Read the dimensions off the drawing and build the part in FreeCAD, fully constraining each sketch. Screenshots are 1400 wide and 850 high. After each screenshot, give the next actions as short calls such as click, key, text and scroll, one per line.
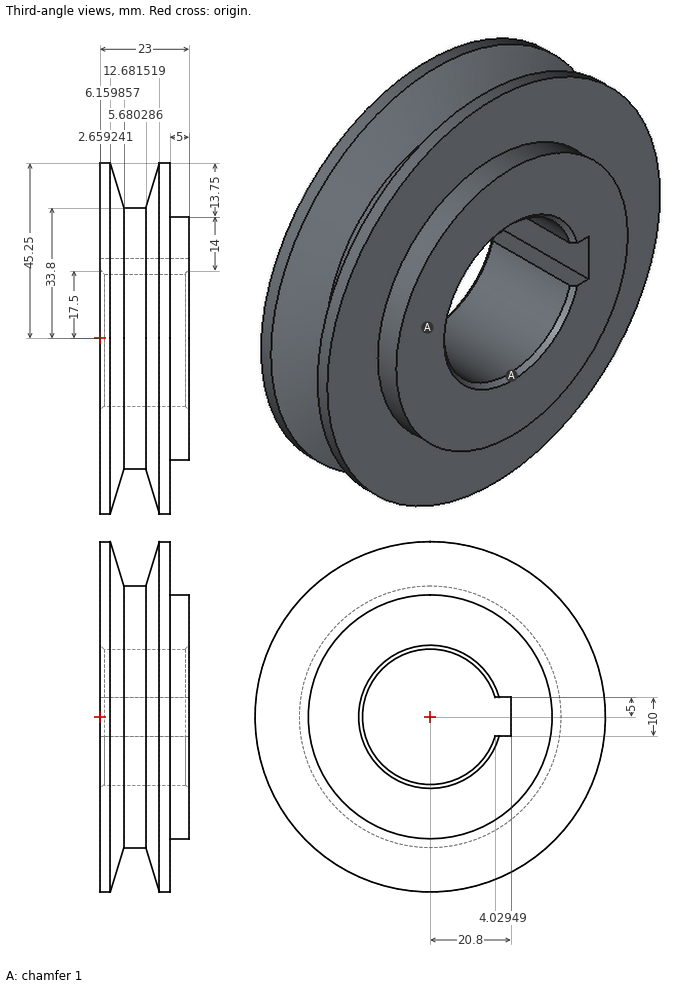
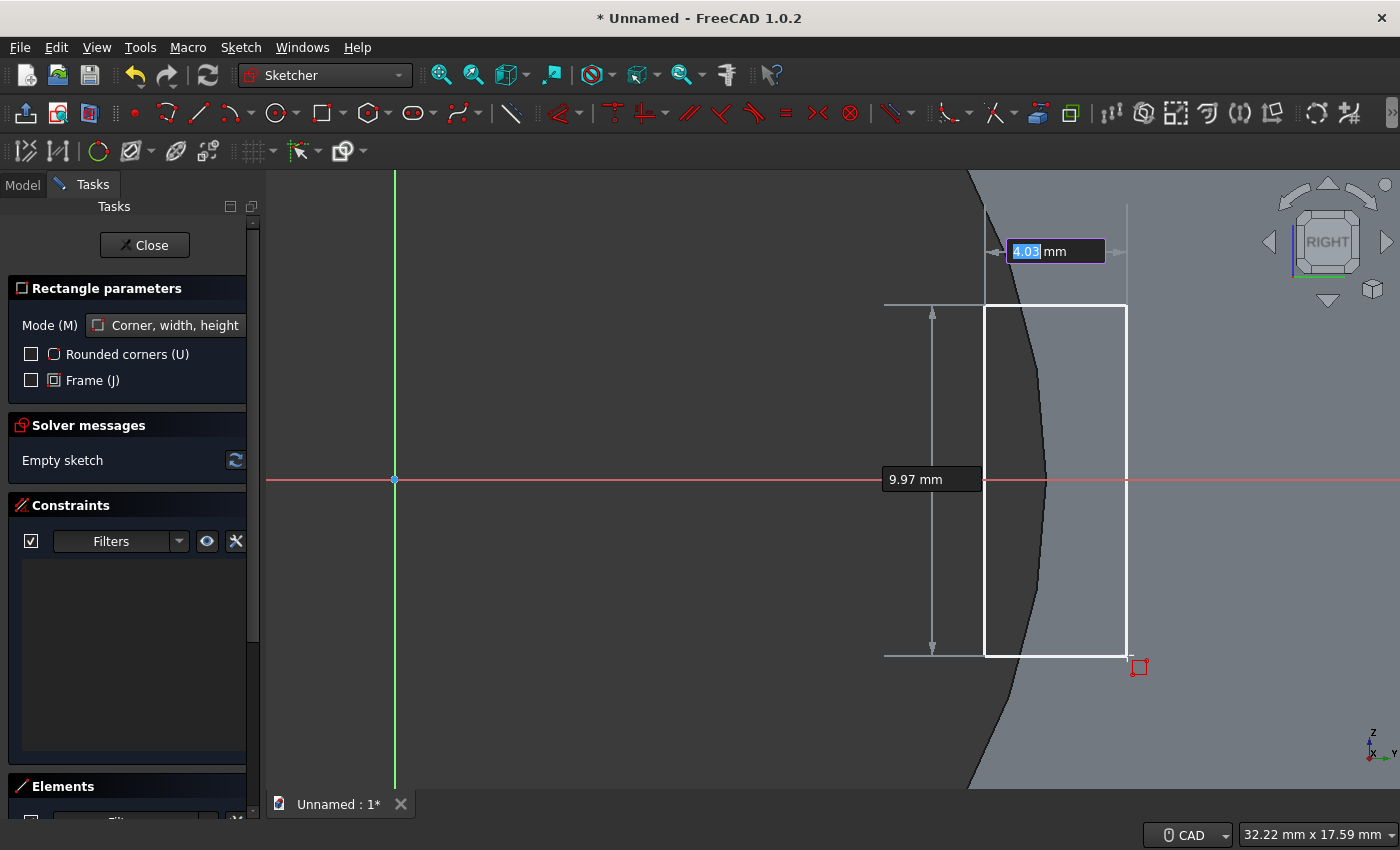
text(4.02949)
key(Tab)
text(10)
key(Return)
key(Escape)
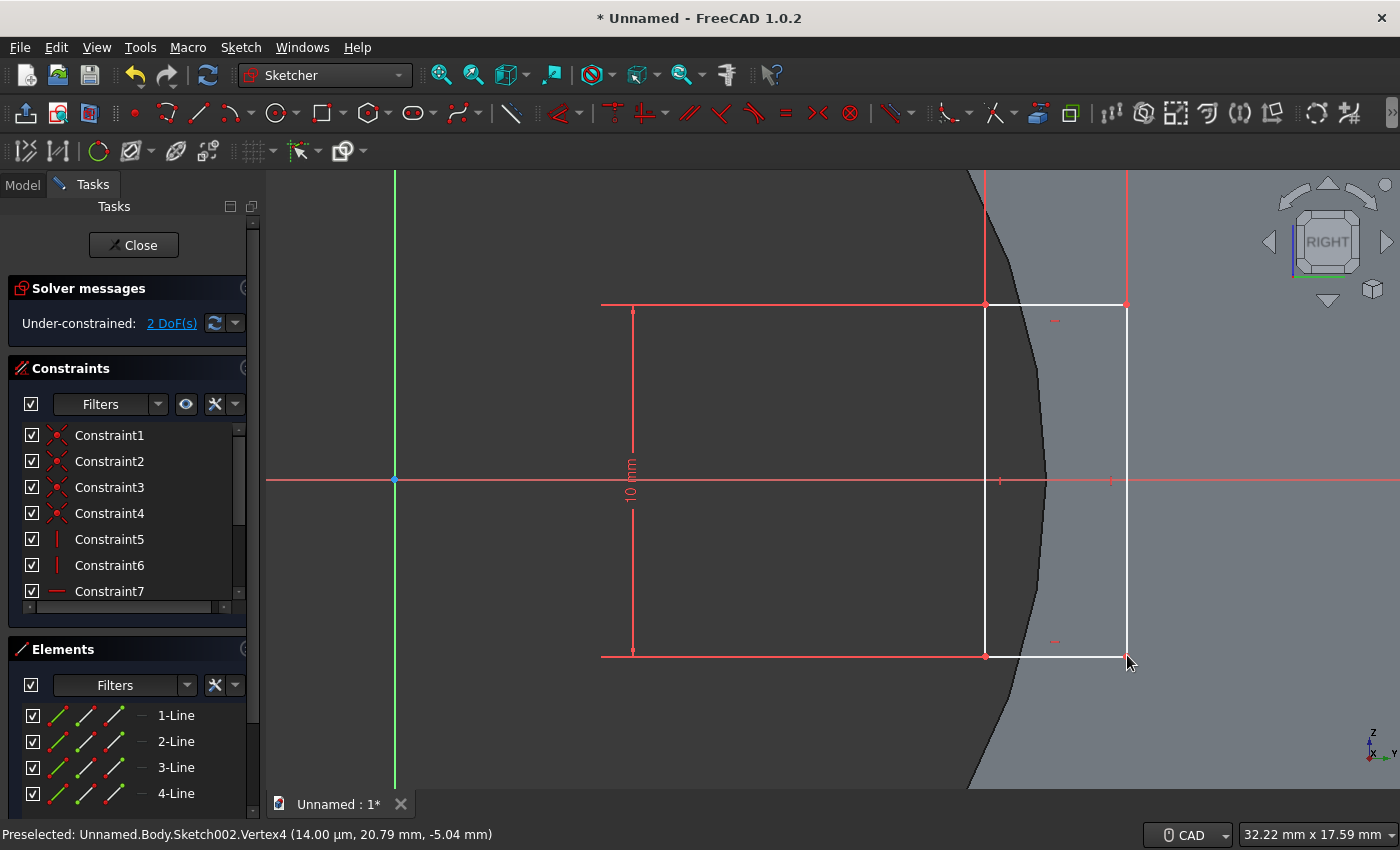
click(558, 114)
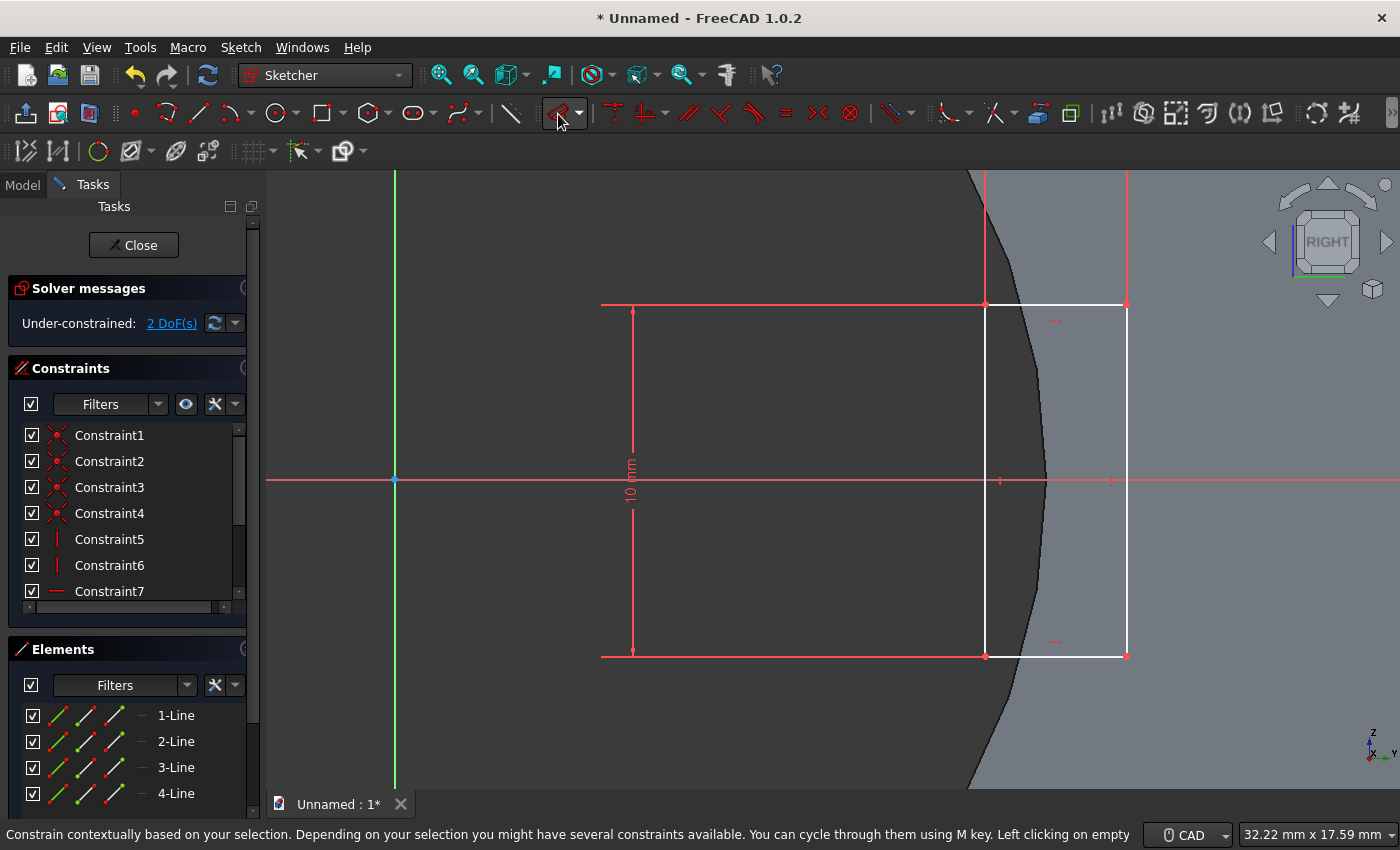
click(985, 305)
click(361, 392)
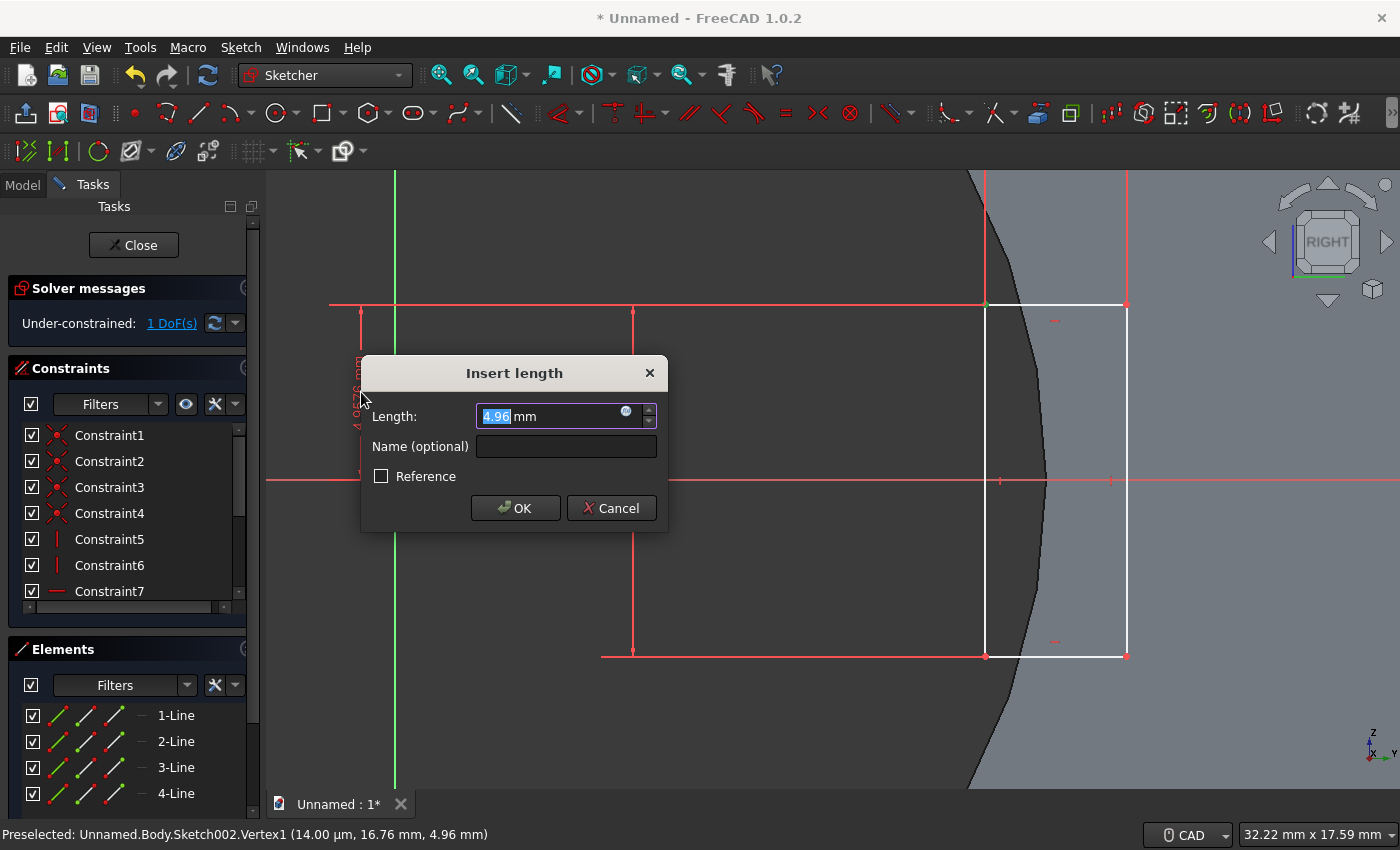
text(5)
key(Return)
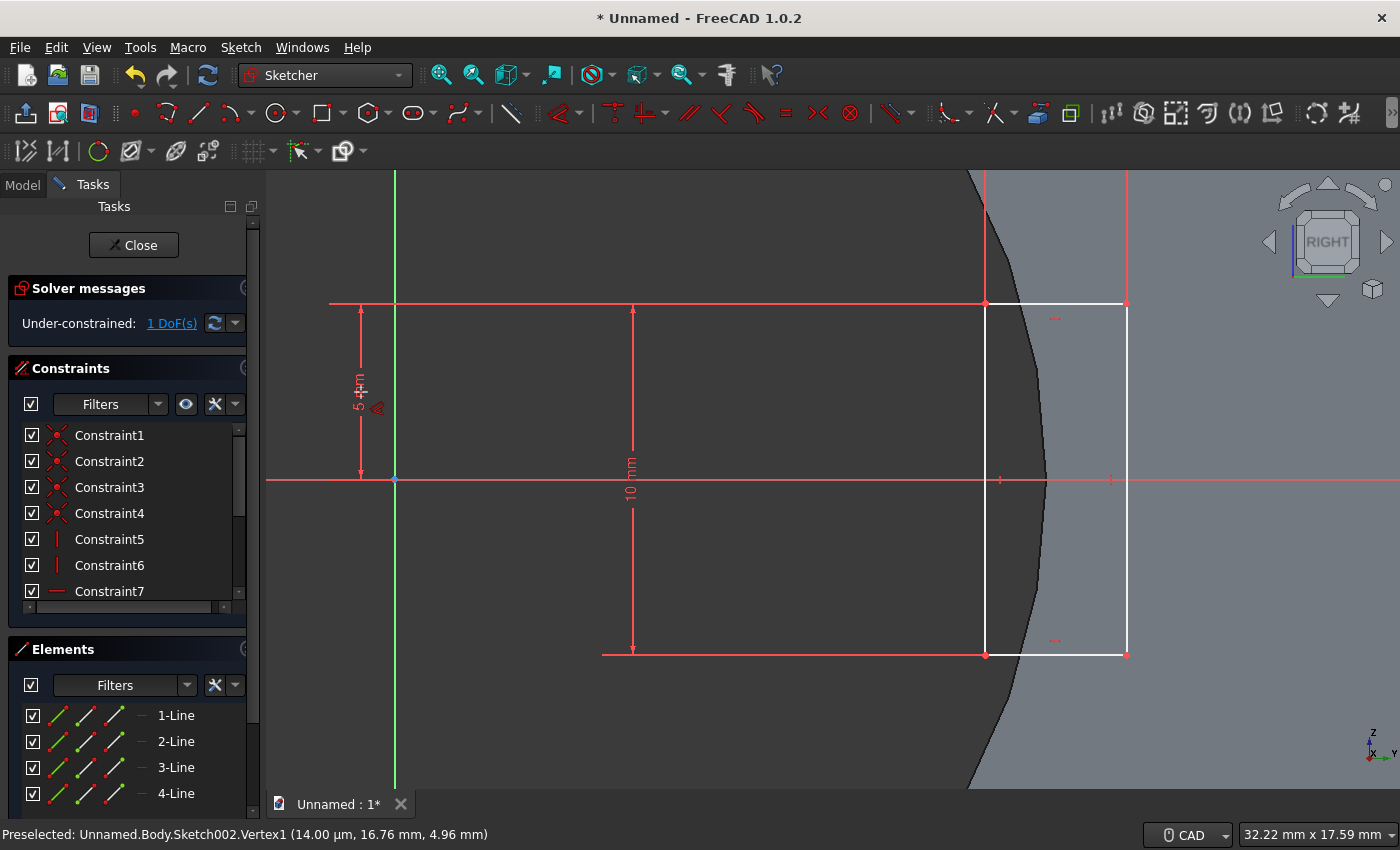
click(1127, 655)
click(761, 689)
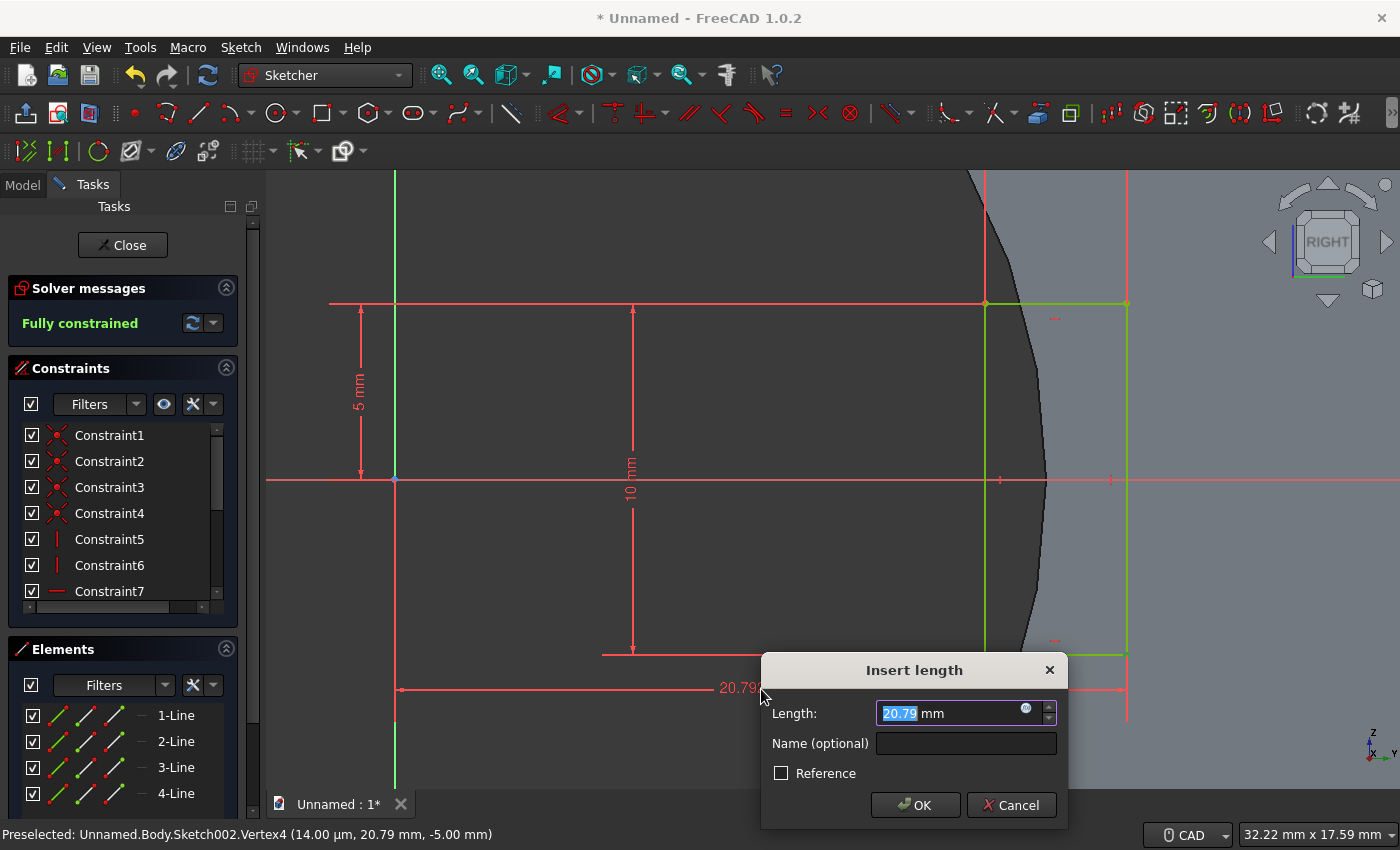
text(20.8)
key(Return)
key(Escape)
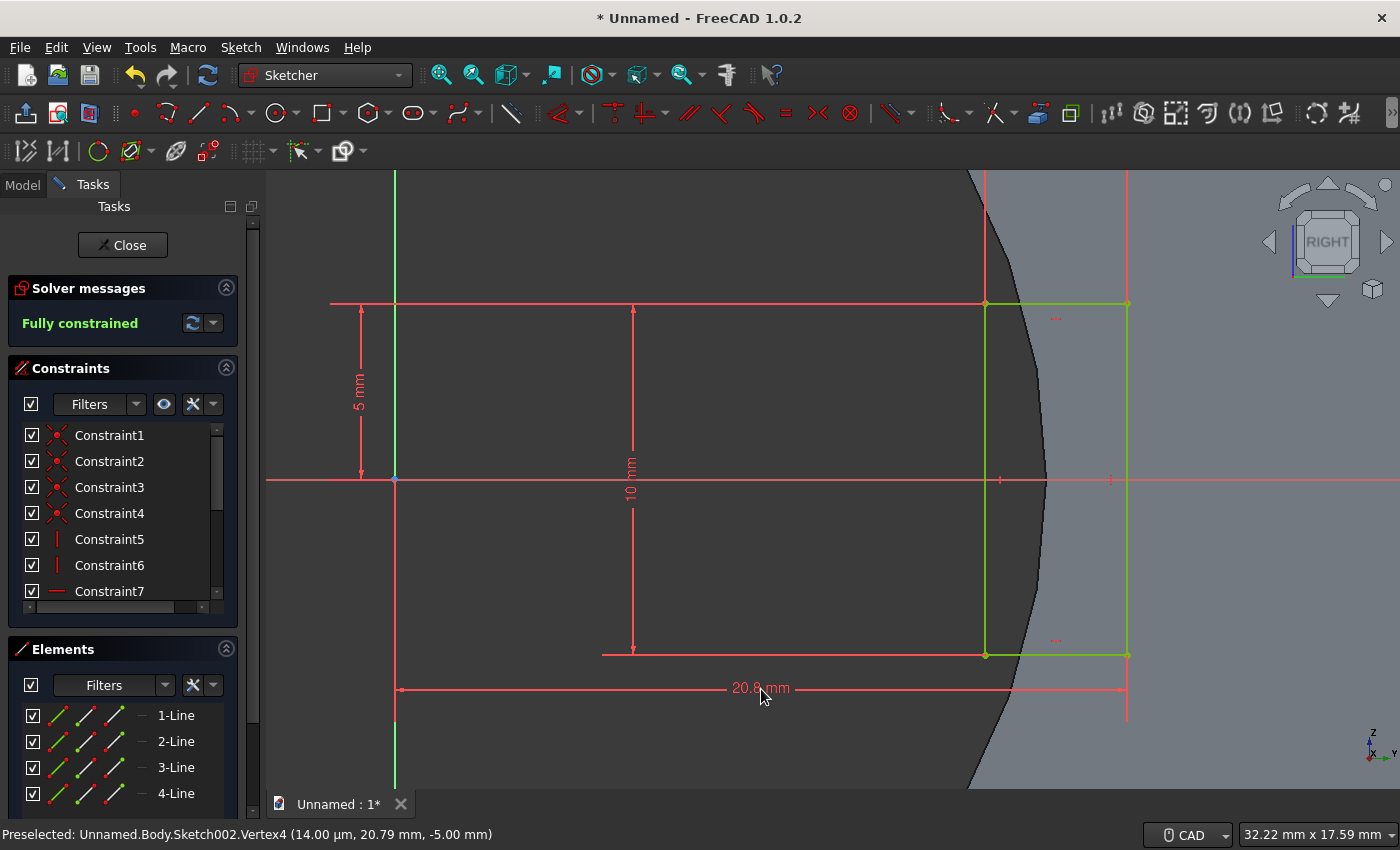
click(123, 245)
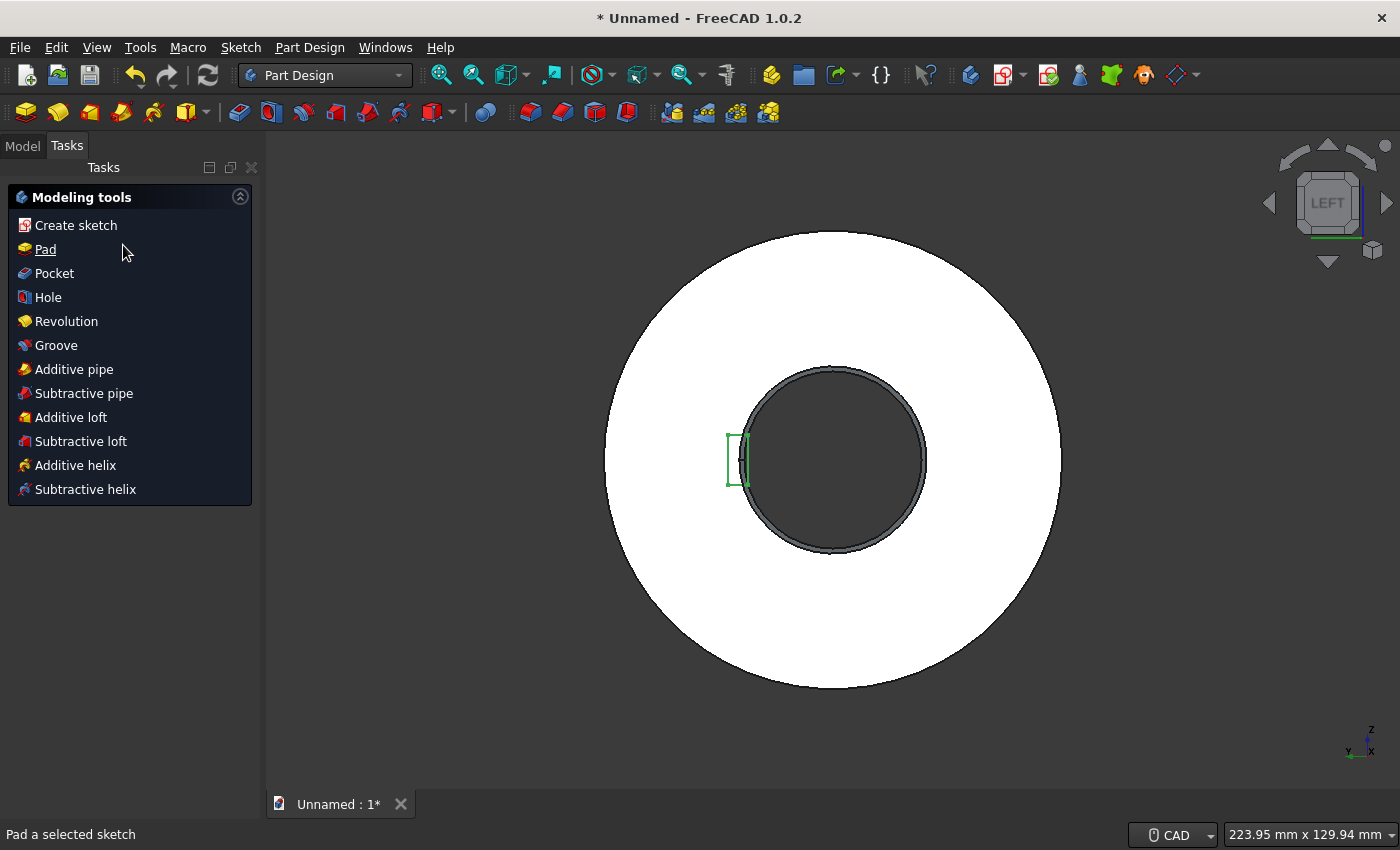
click(240, 112)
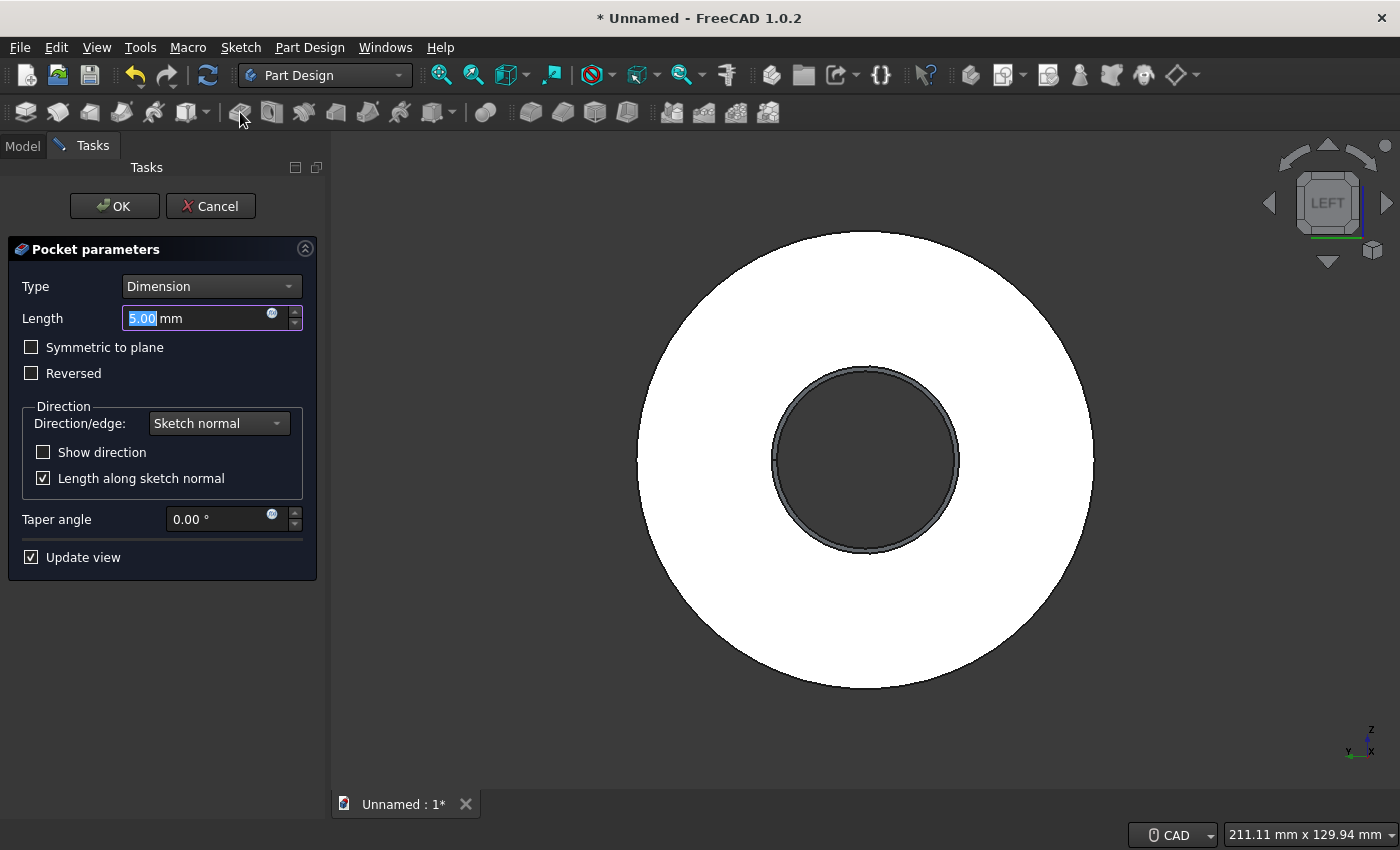
click(212, 286)